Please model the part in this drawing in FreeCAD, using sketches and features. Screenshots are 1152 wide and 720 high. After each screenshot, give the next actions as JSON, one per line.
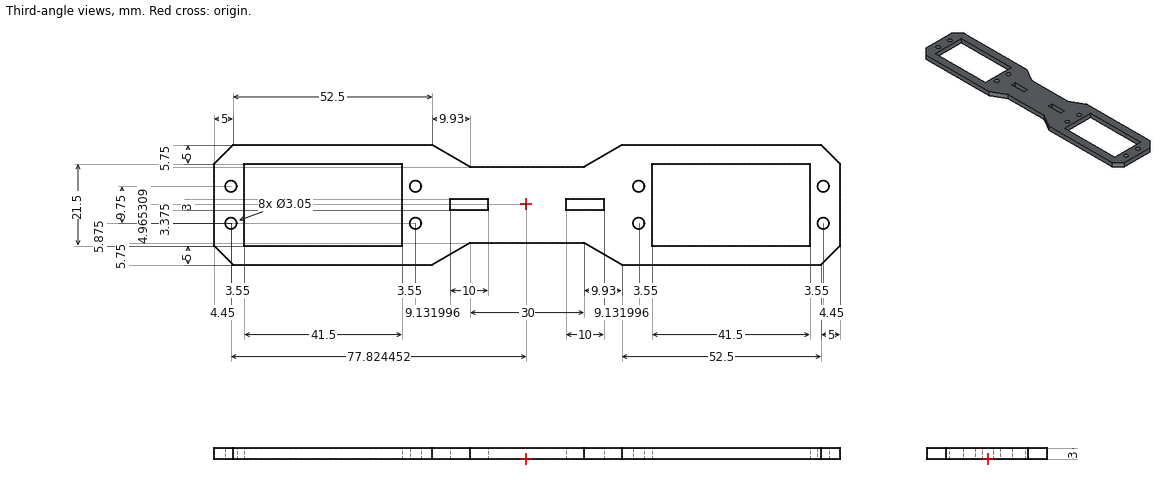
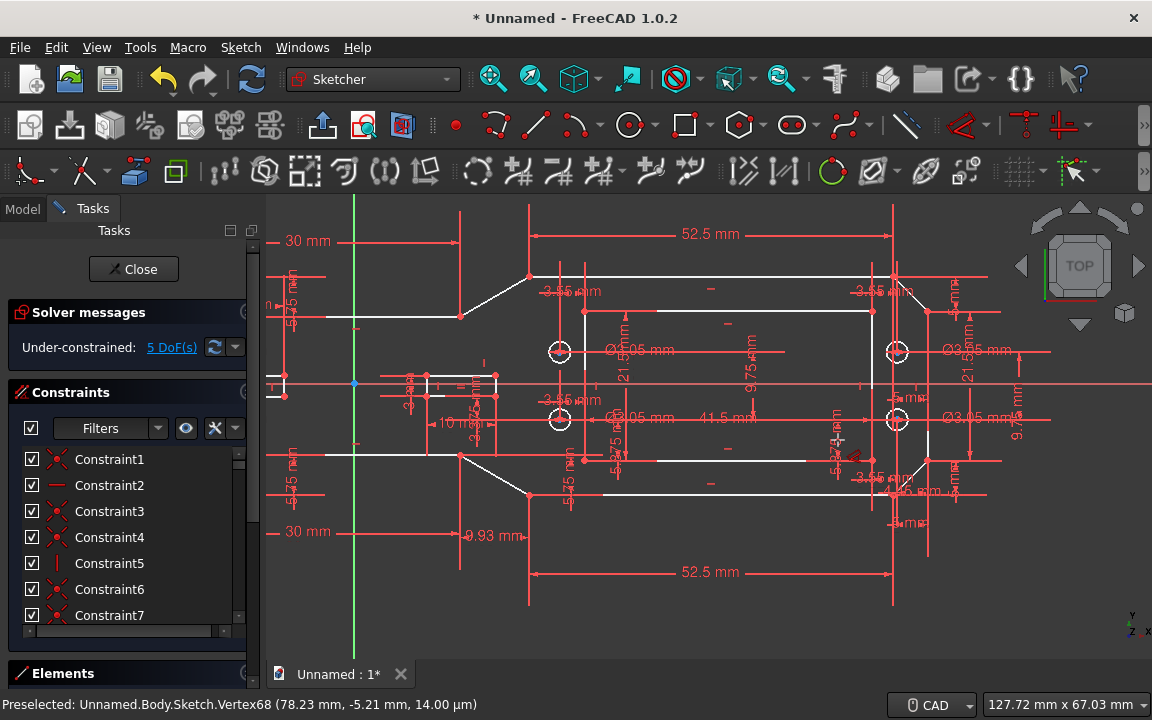
{"action": "left_click", "coordinate": [928, 461]}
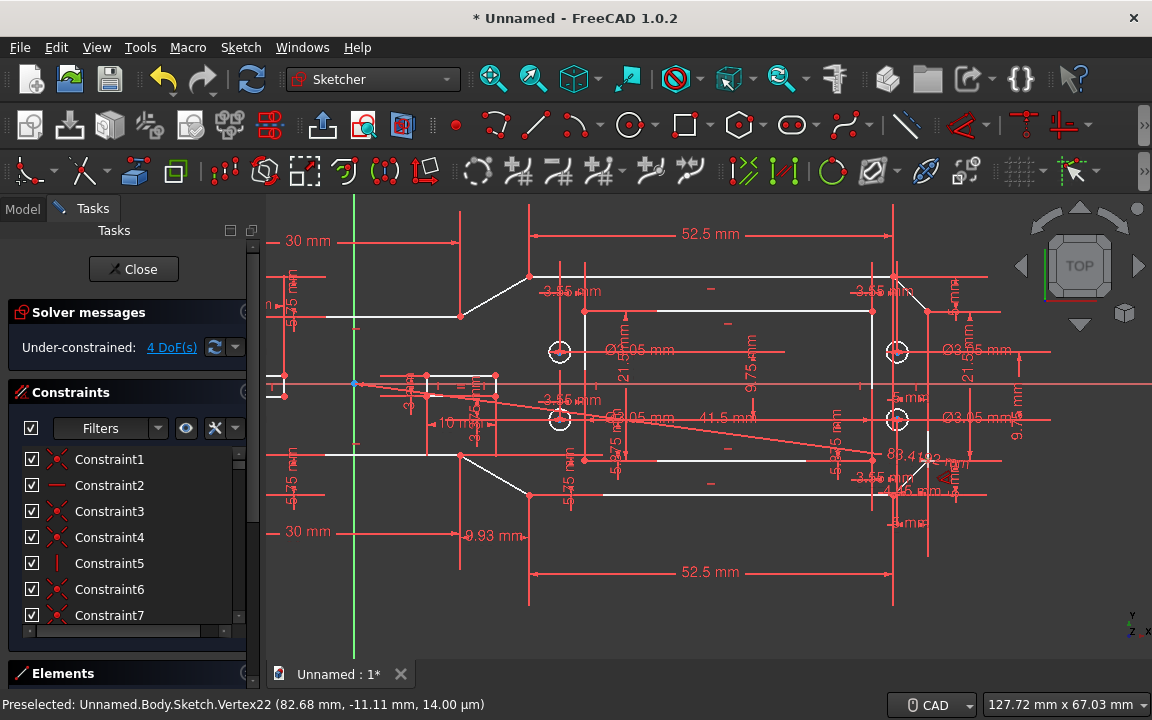
{"action": "left_click", "coordinate": [897, 420]}
{"action": "left_click", "coordinate": [962, 440]}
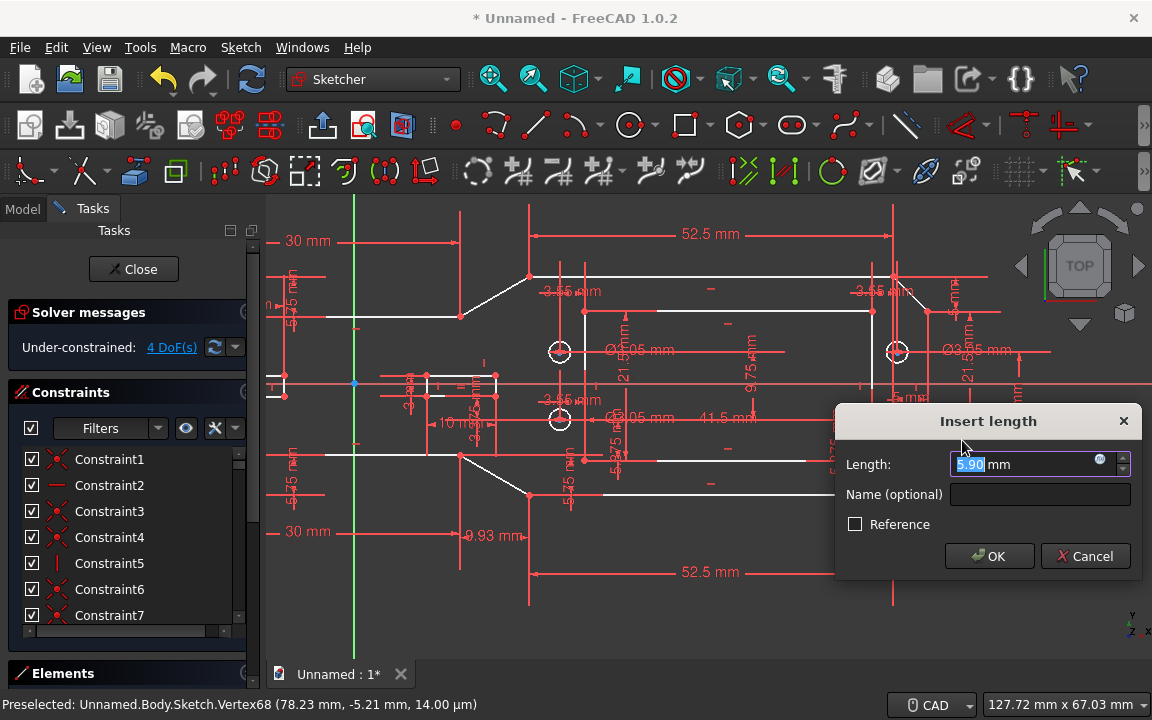
{"action": "type", "text": "5.875"}
{"action": "key", "text": "Return"}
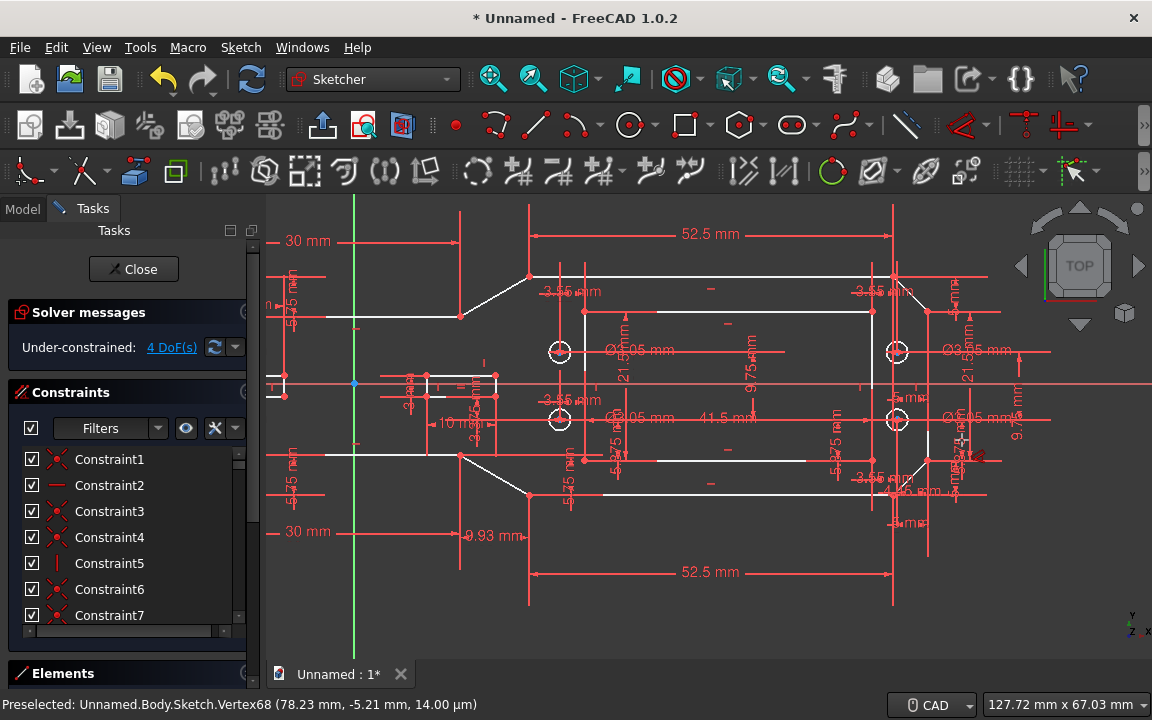
{"action": "scroll", "coordinate": [873, 461], "scroll_direction": "down", "scroll_amount": 4}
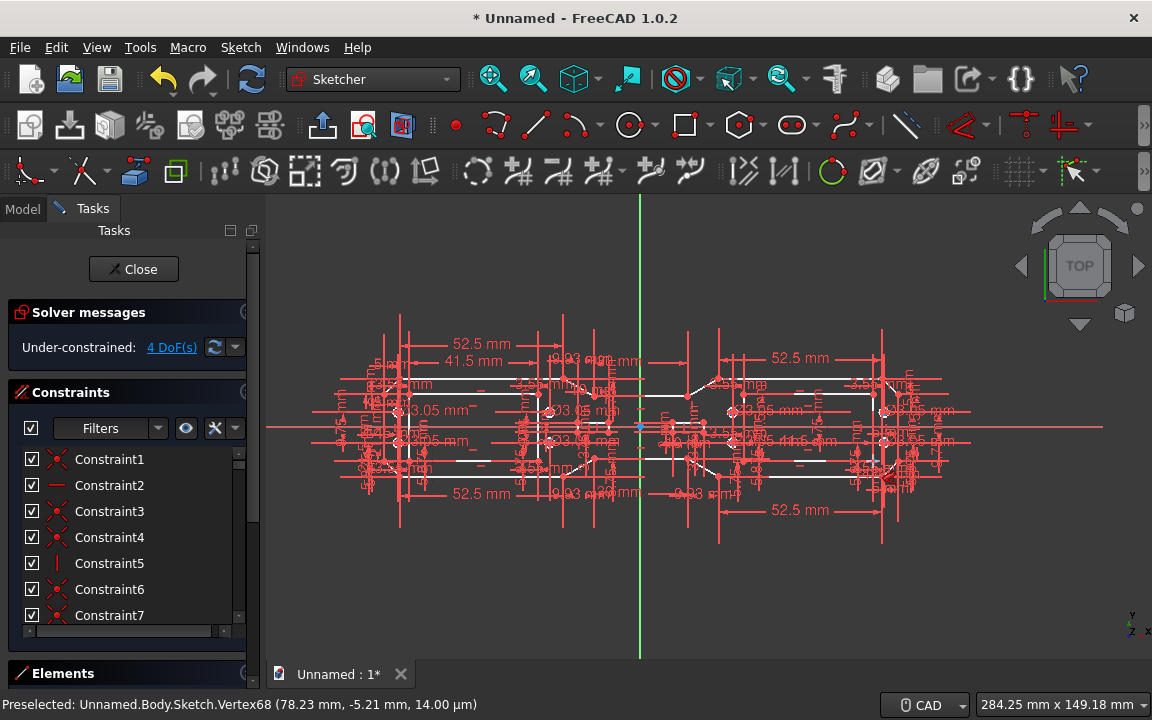
{"action": "left_click", "coordinate": [398, 443]}
{"action": "left_click", "coordinate": [519, 525]}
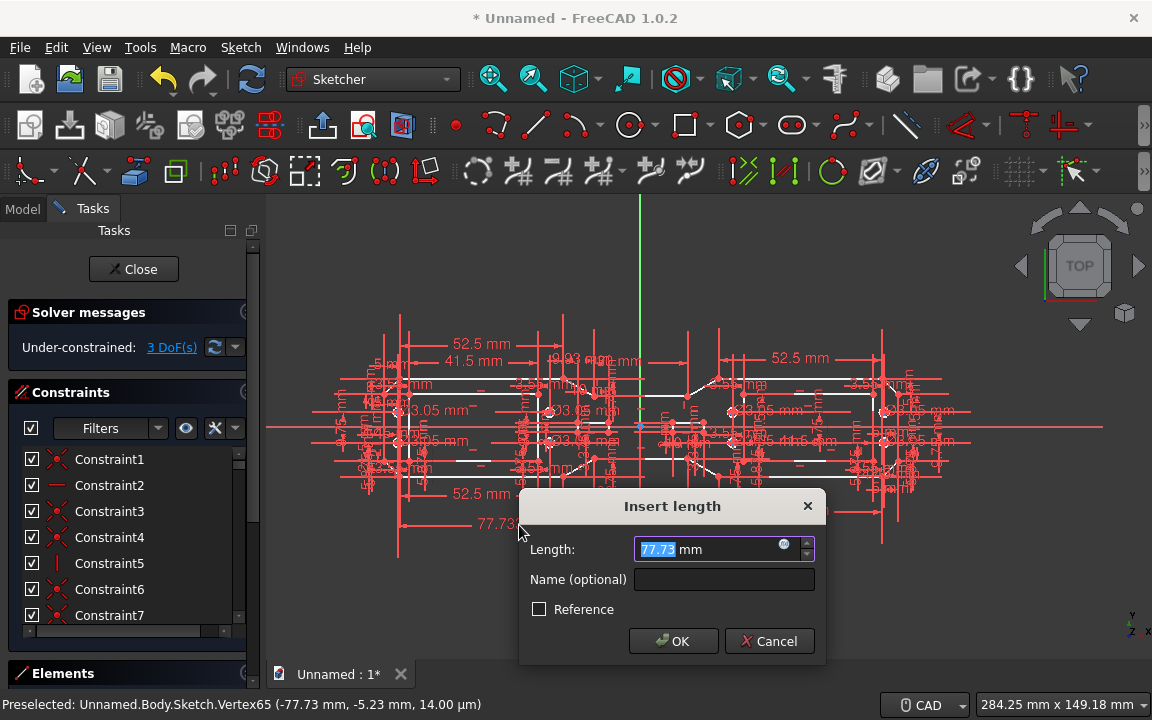
{"action": "type", "text": "77.824452"}
{"action": "key", "text": "Return"}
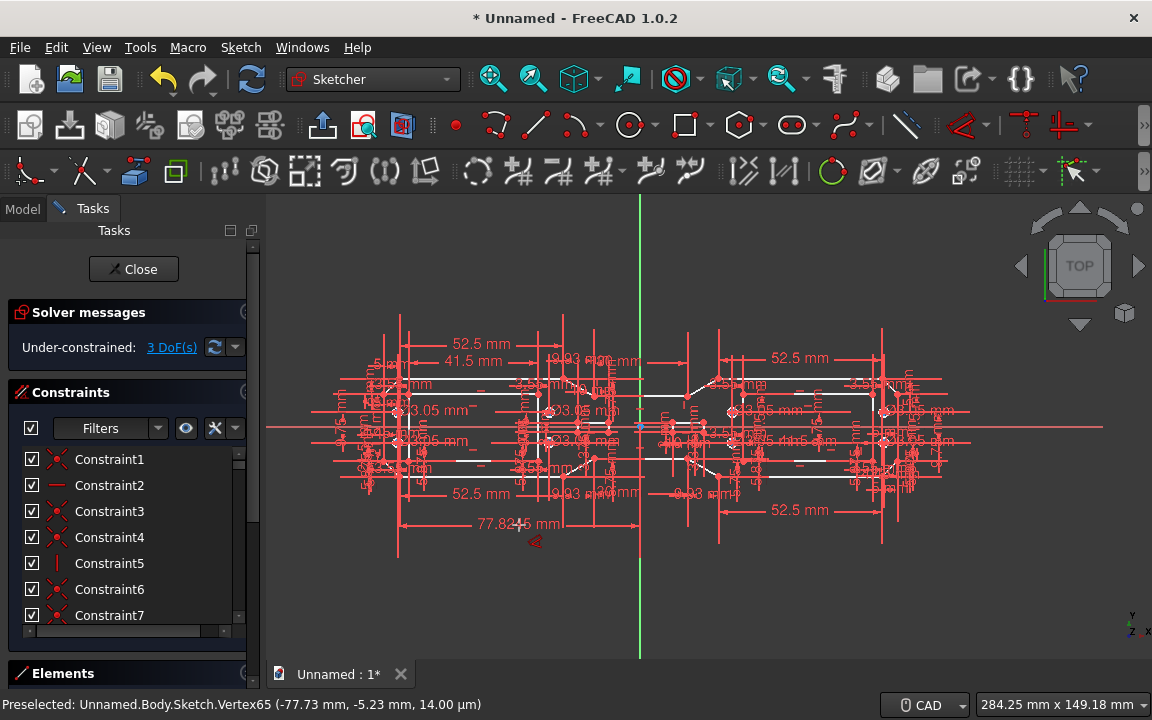
{"action": "scroll", "coordinate": [578, 432], "scroll_direction": "up", "scroll_amount": 2}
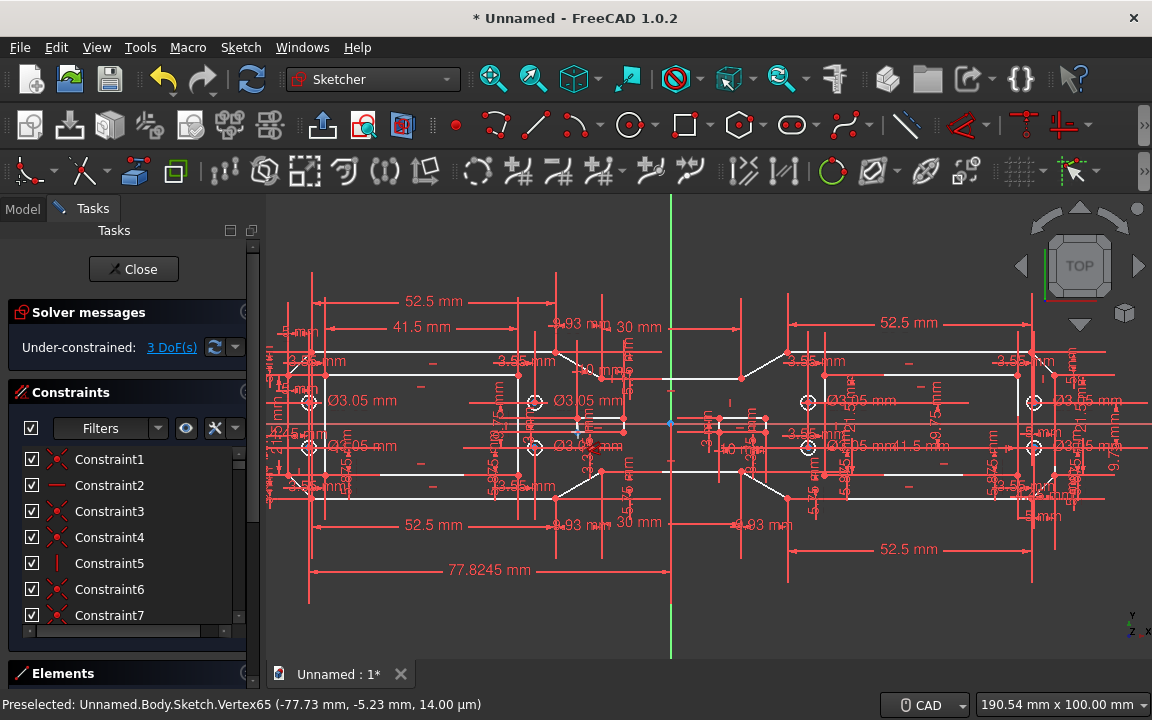
{"action": "left_click", "coordinate": [577, 432]}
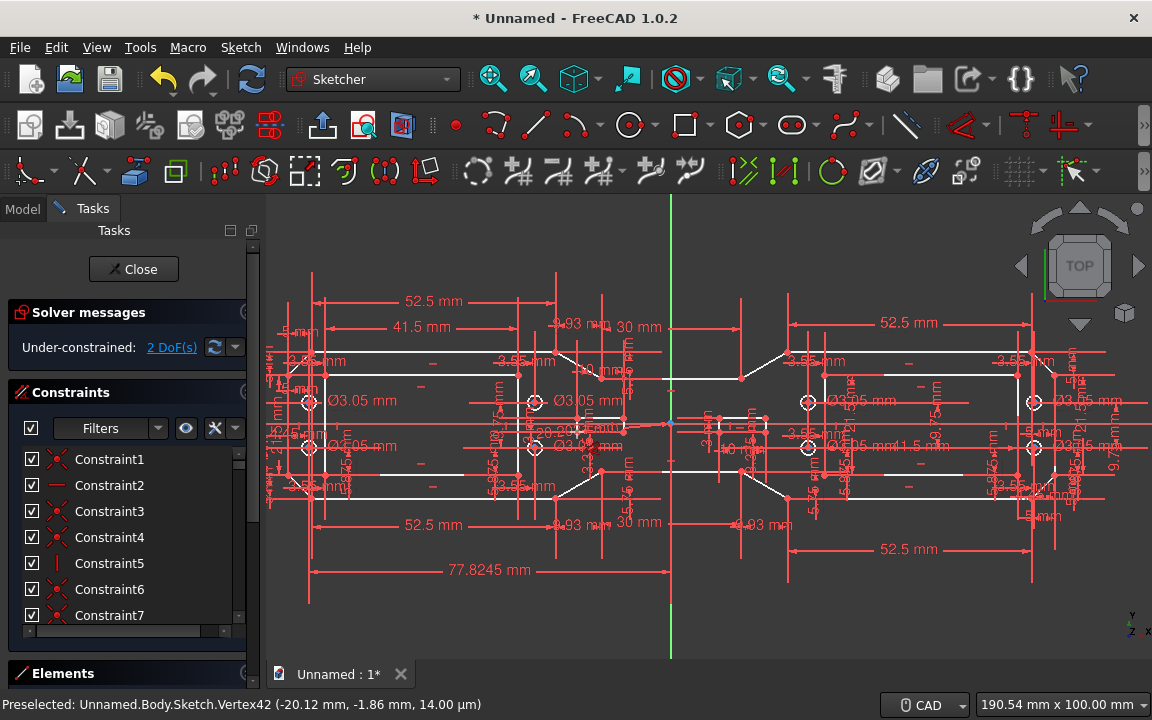
{"action": "left_click", "coordinate": [535, 448]}
{"action": "left_click", "coordinate": [566, 554]}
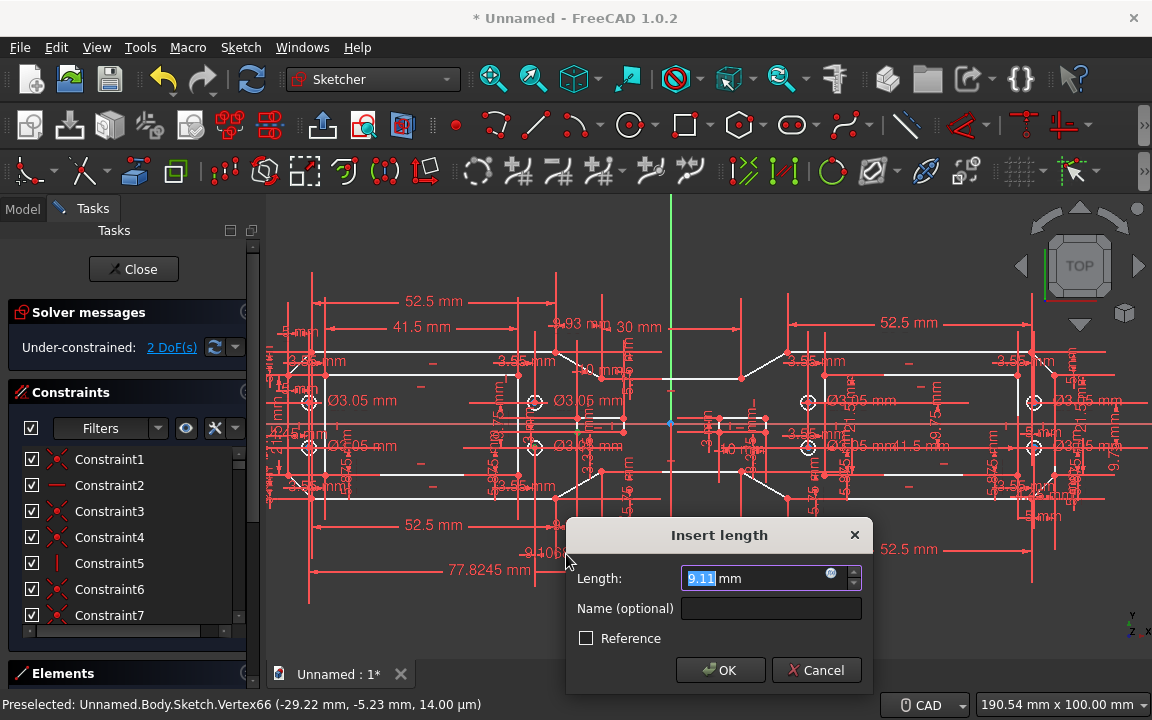
{"action": "type", "text": "9.131996"}
{"action": "key", "text": "Return"}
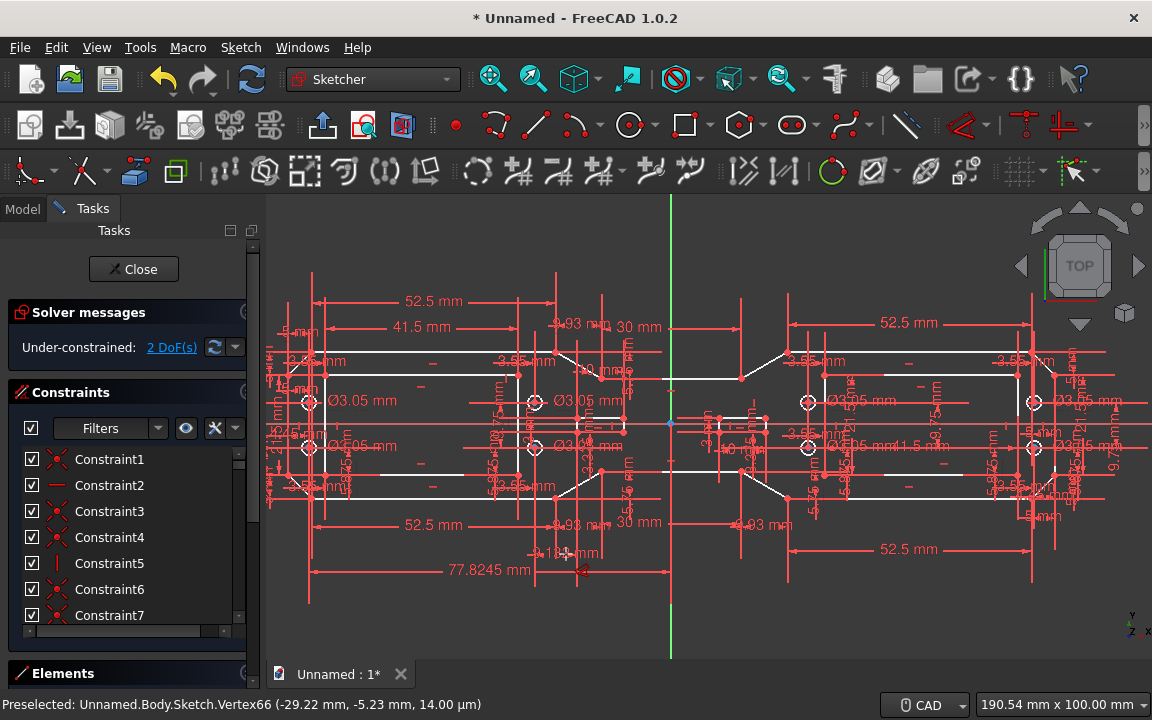
{"action": "left_click", "coordinate": [766, 432]}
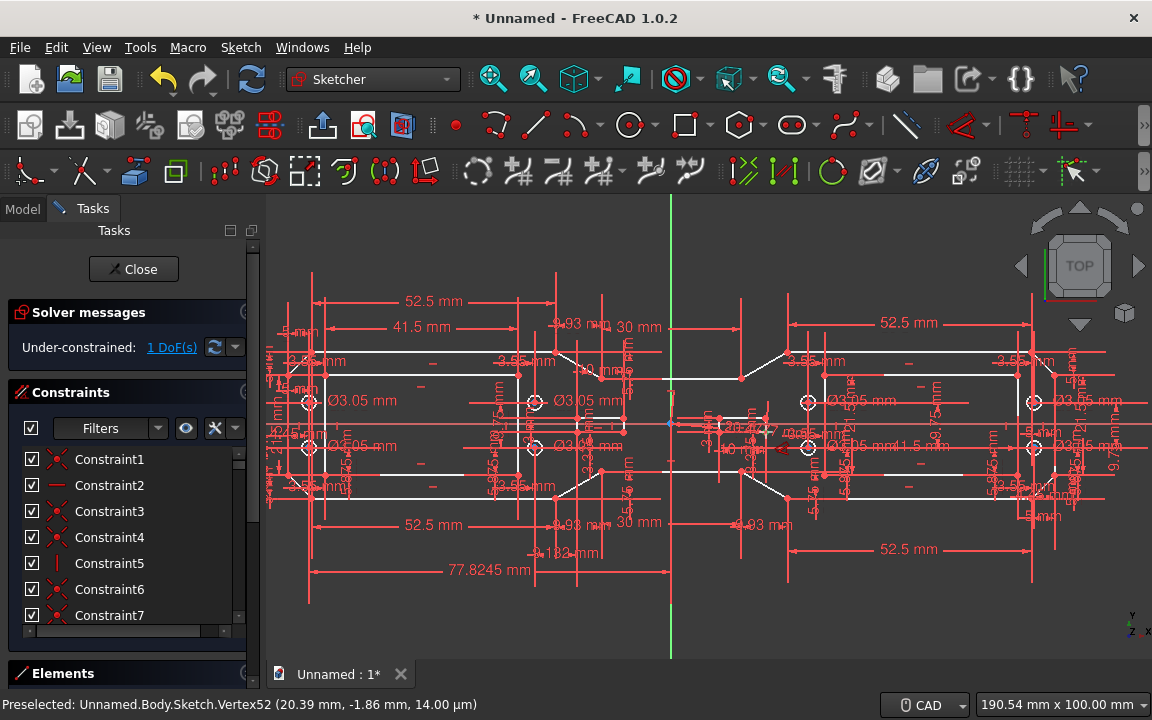
{"action": "left_click", "coordinate": [808, 448]}
{"action": "left_click", "coordinate": [777, 398]}